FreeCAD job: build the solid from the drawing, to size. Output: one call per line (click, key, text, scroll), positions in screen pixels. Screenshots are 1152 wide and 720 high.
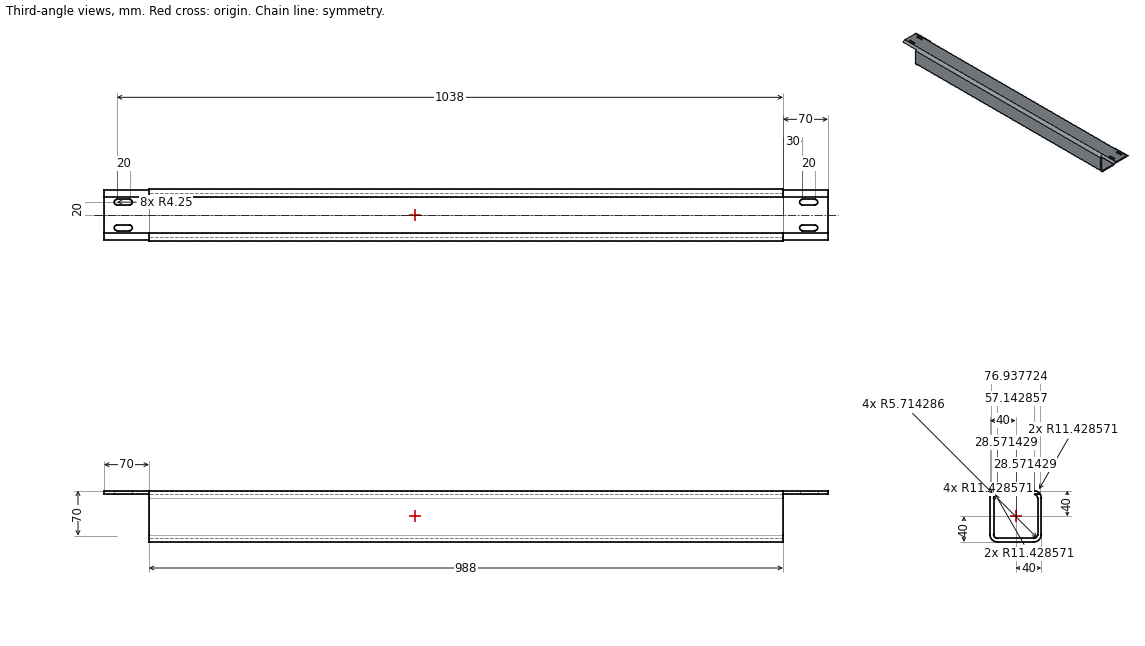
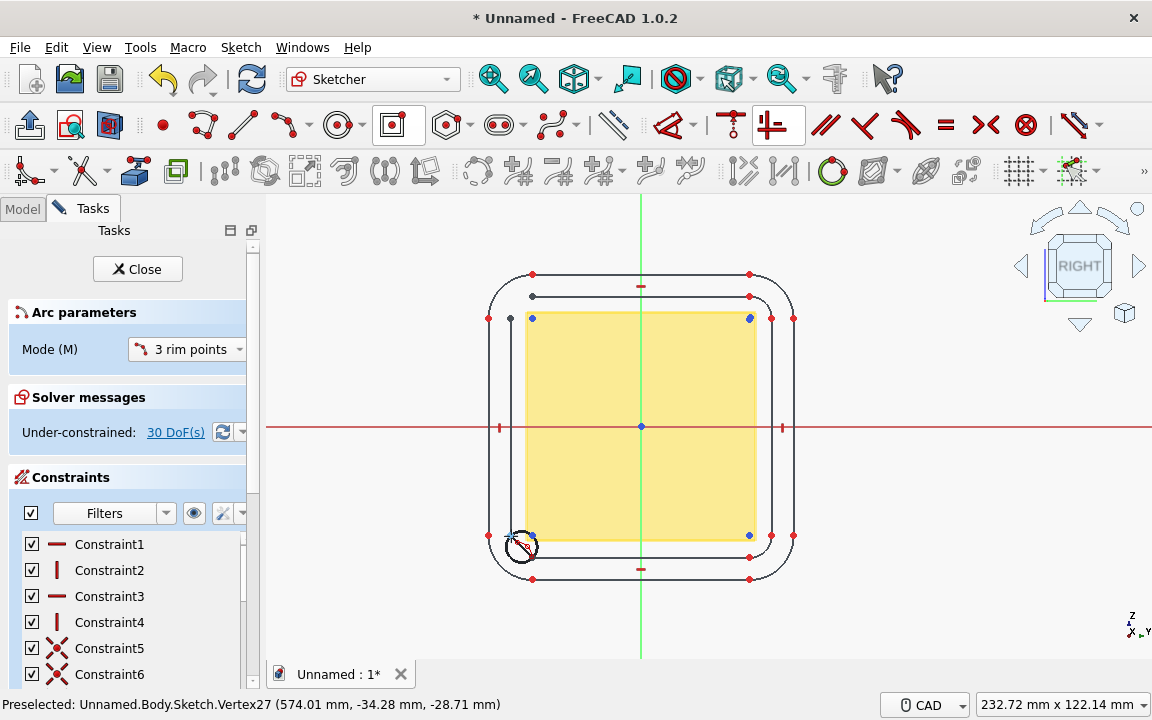
scroll(517, 551, up, 5)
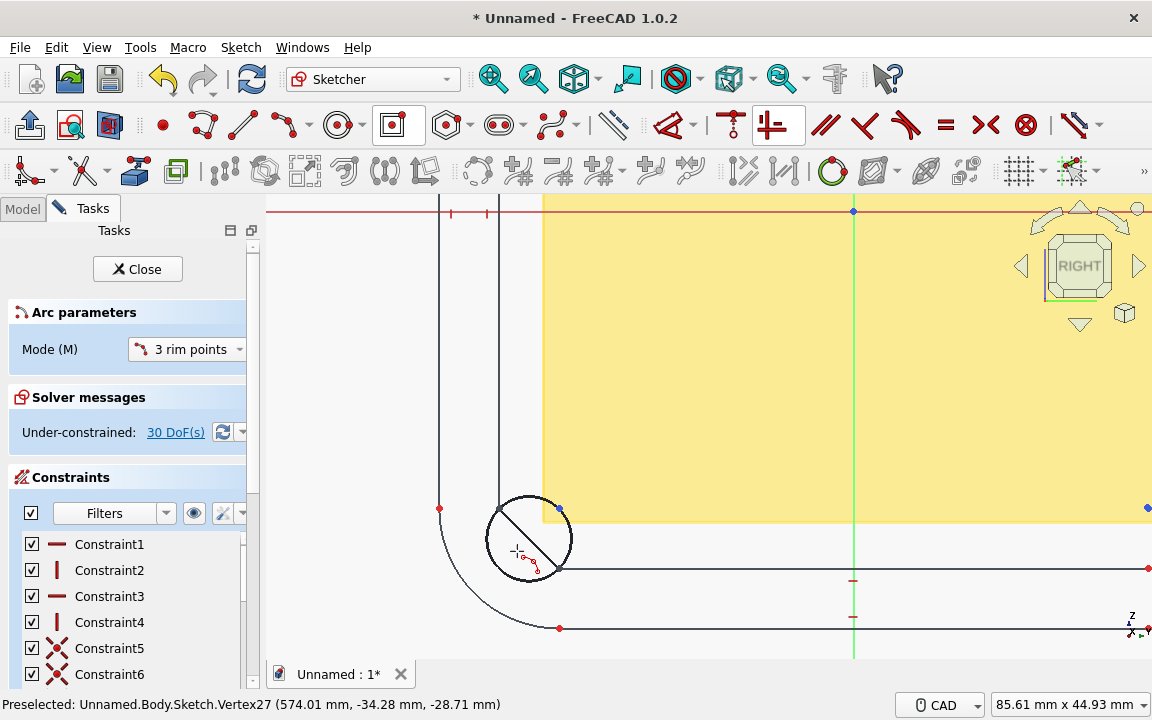
click(516, 549)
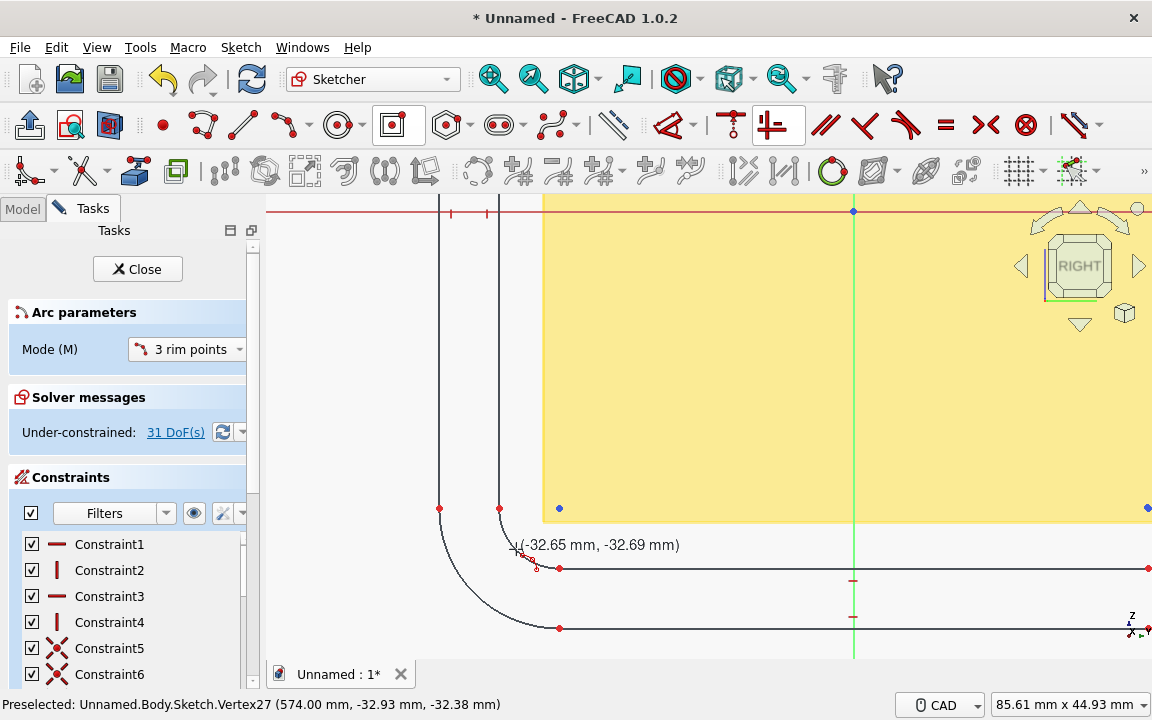
scroll(516, 551, down, 5)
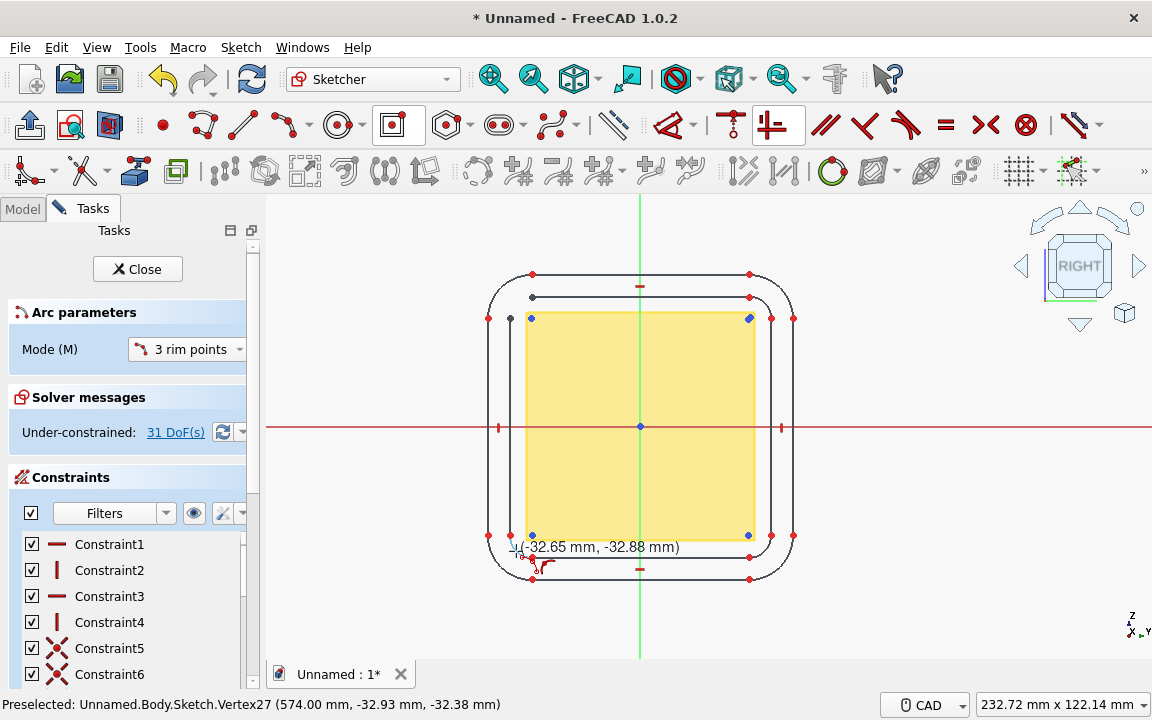
click(510, 319)
click(532, 297)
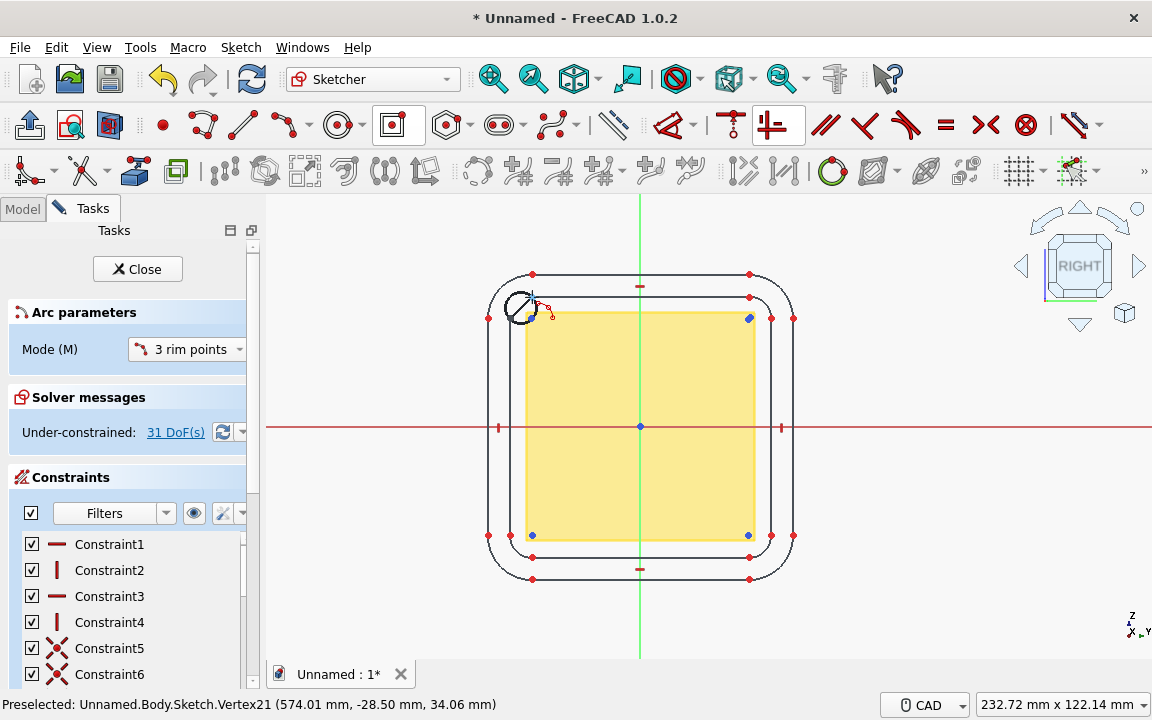
scroll(516, 303, up, 5)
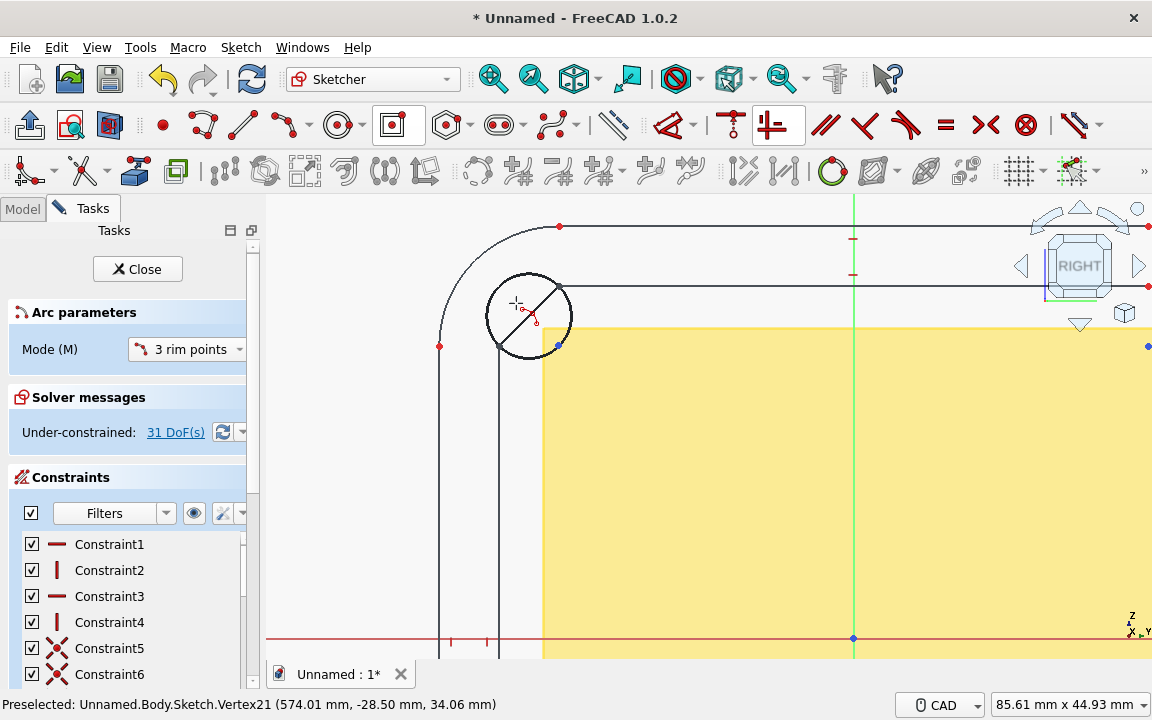
click(516, 301)
key(Escape)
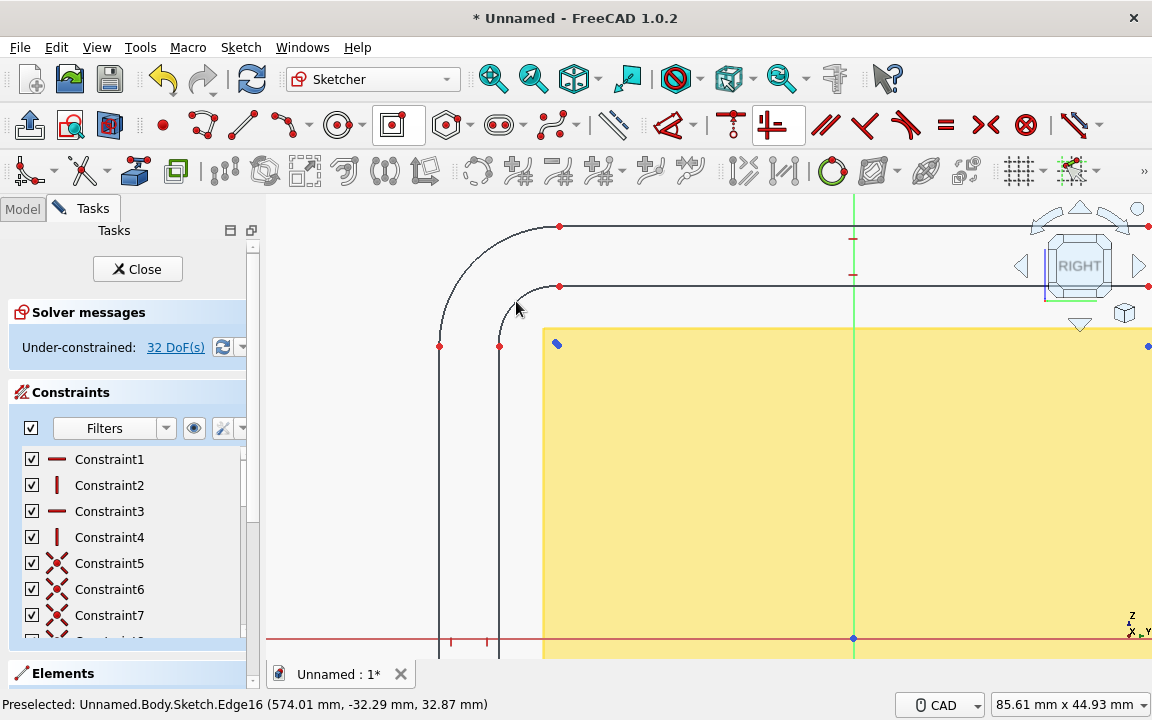
scroll(516, 303, down, 5)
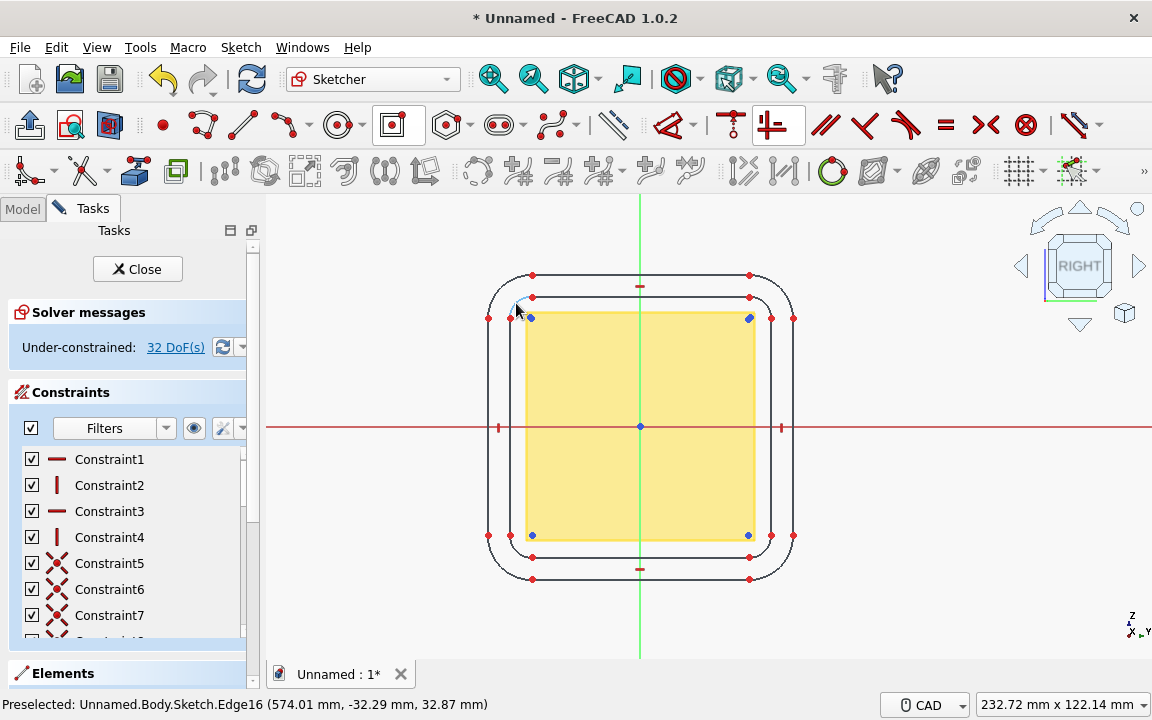
click(597, 580)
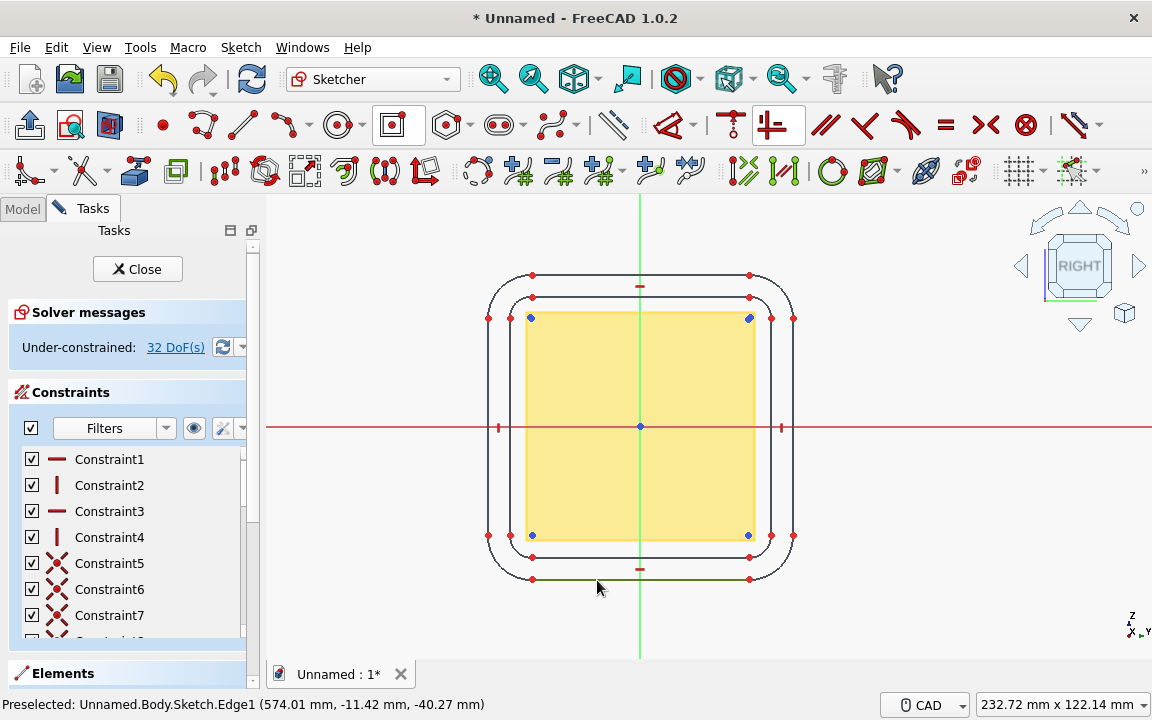
click(769, 575)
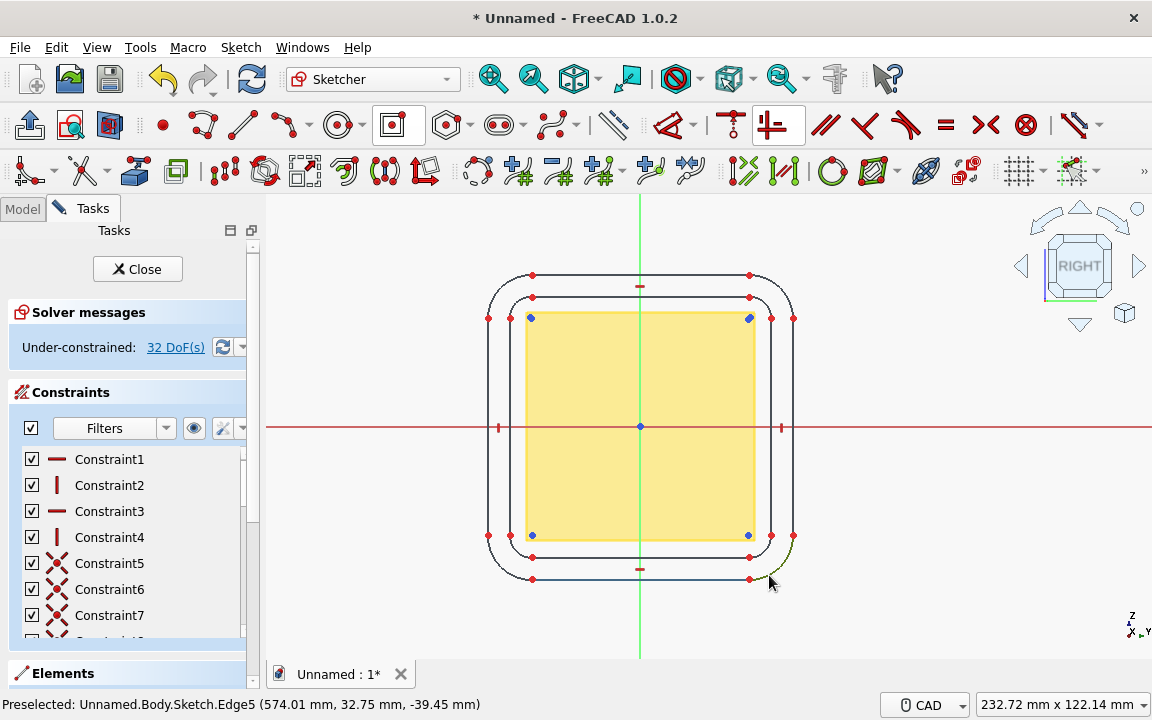
key(t)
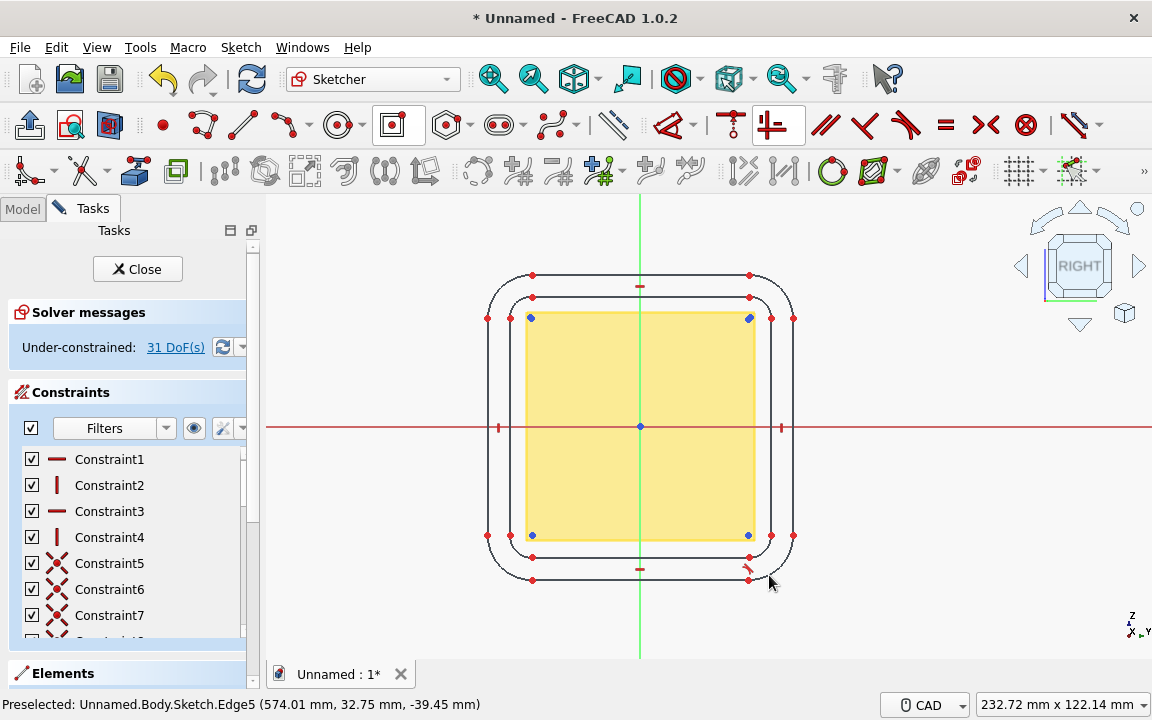
click(597, 580)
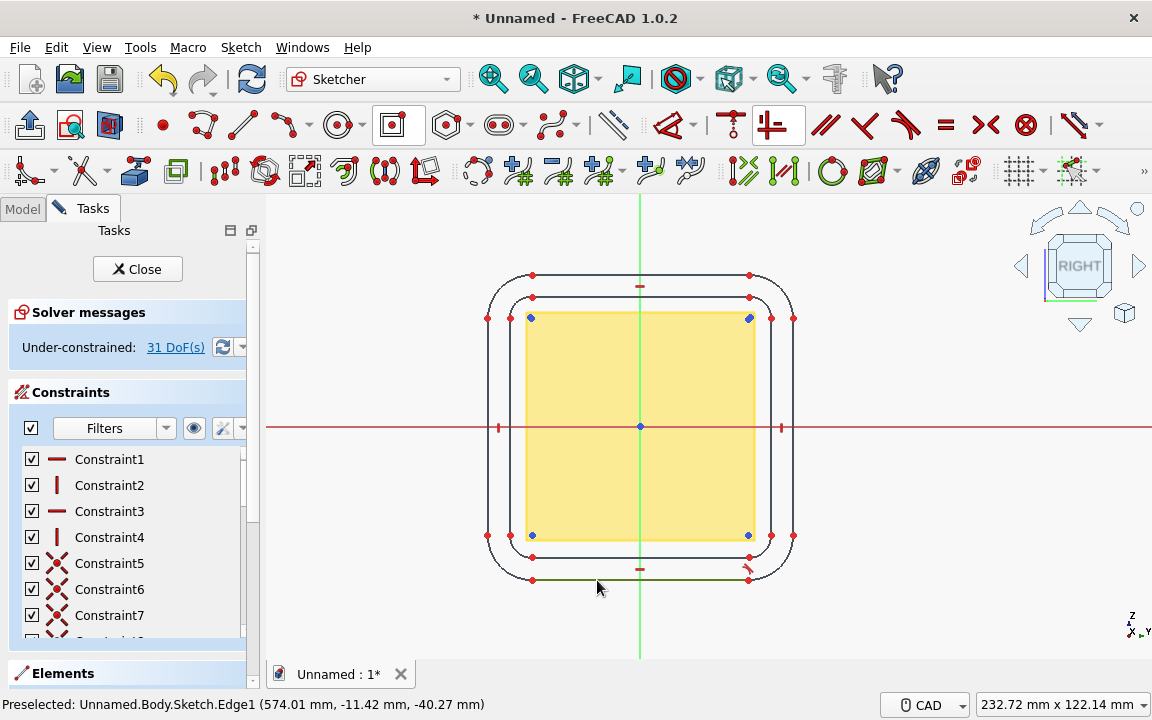
click(493, 556)